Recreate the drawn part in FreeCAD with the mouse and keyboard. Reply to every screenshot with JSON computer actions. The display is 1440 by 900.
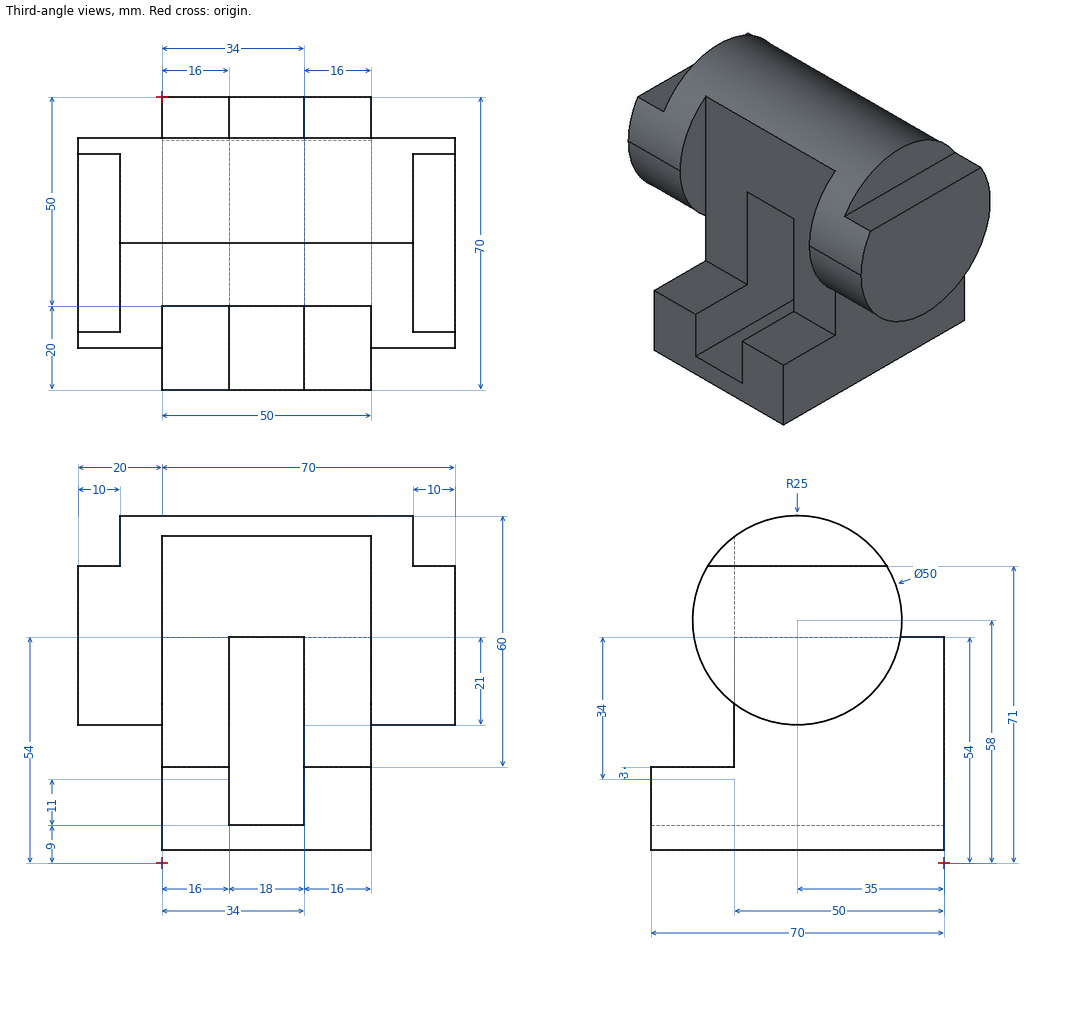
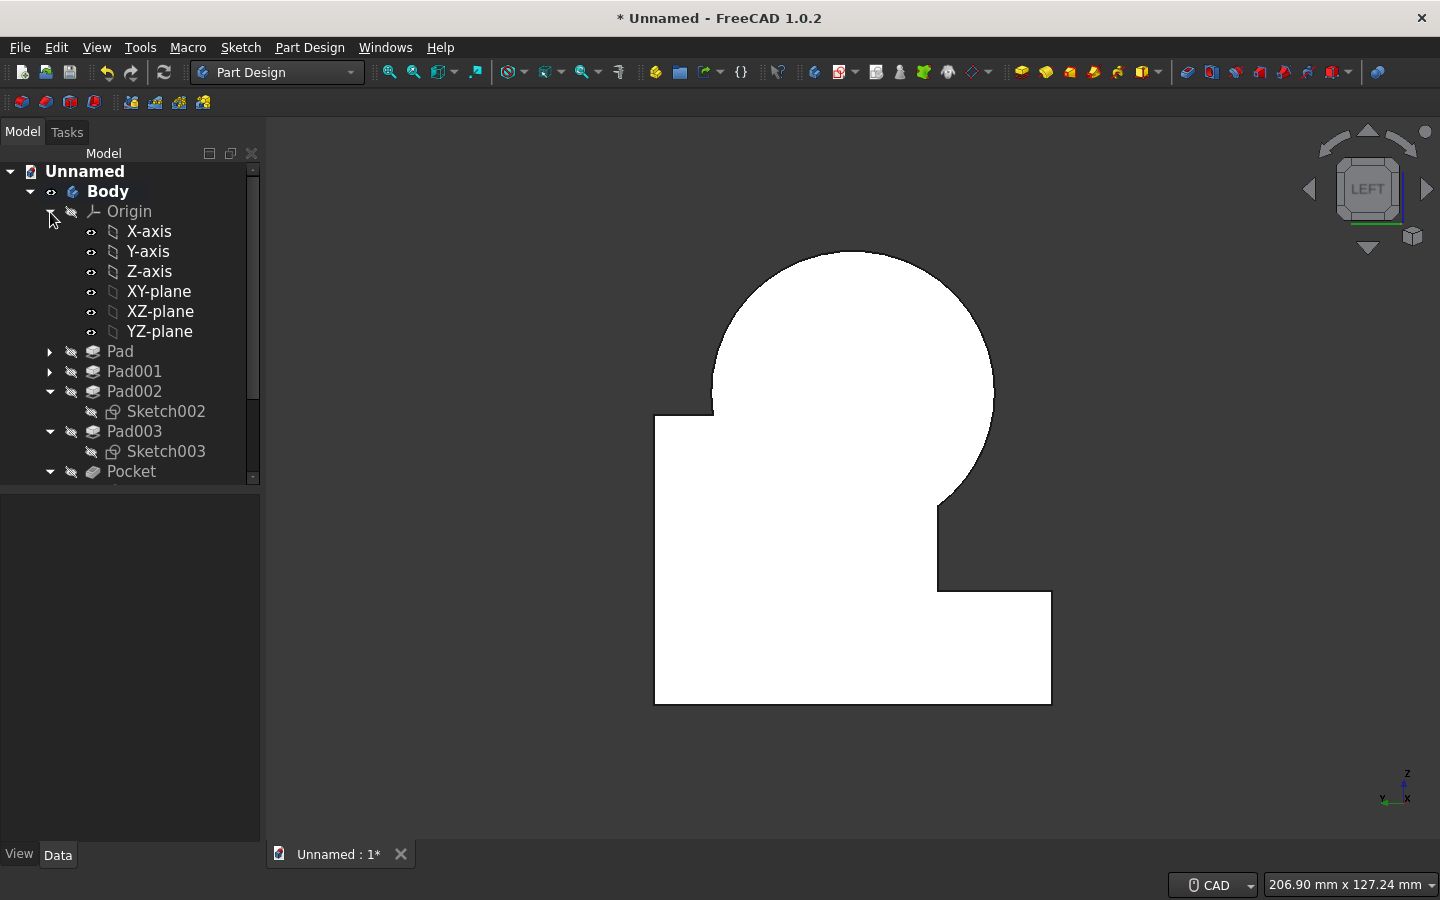
{"action": "left_click", "coordinate": [136, 332]}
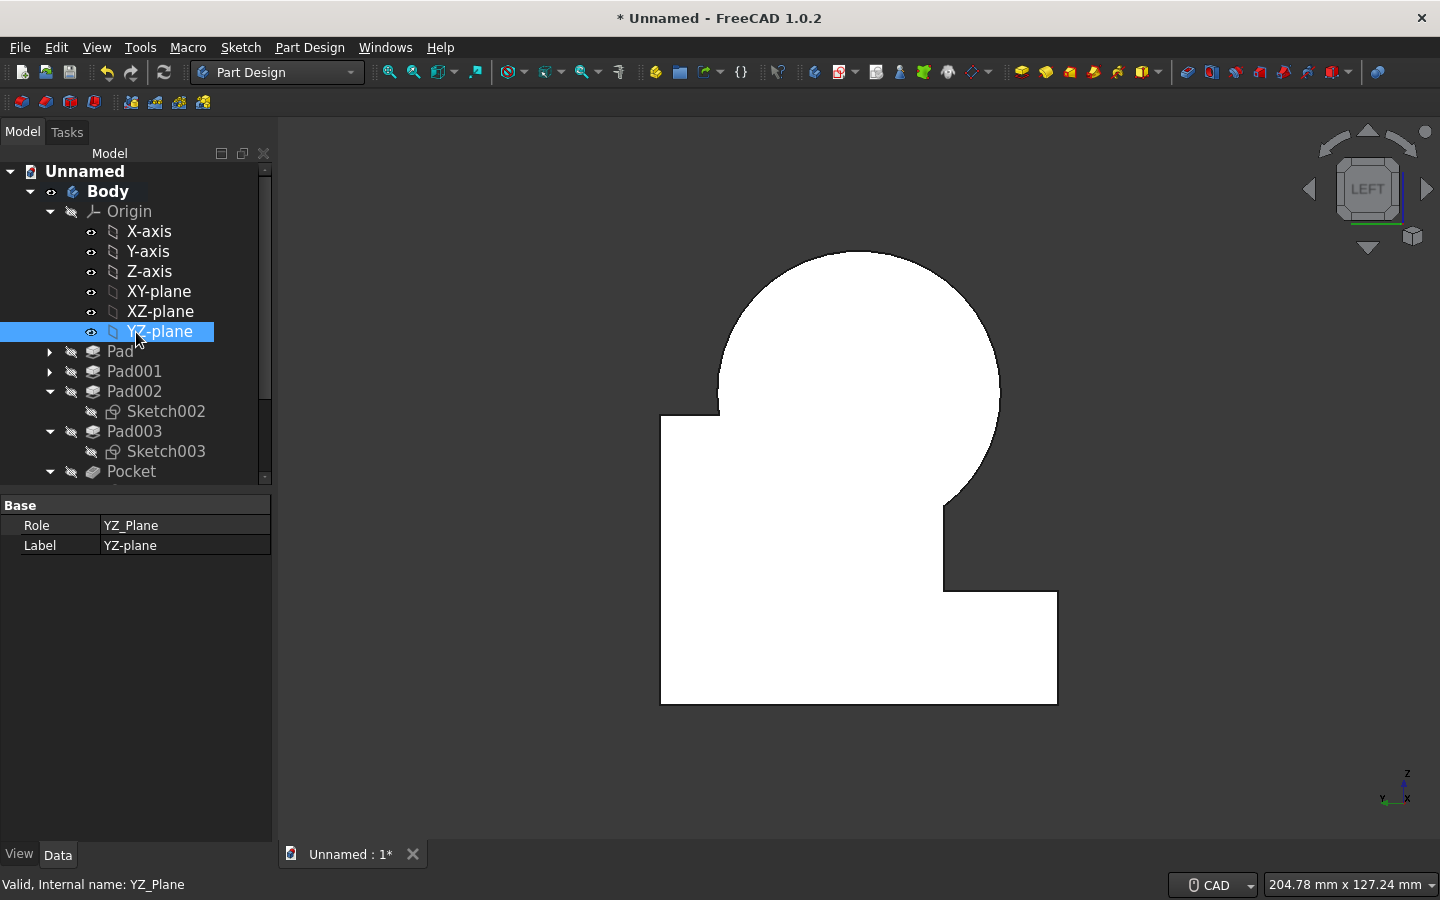
{"action": "left_click", "coordinate": [972, 72]}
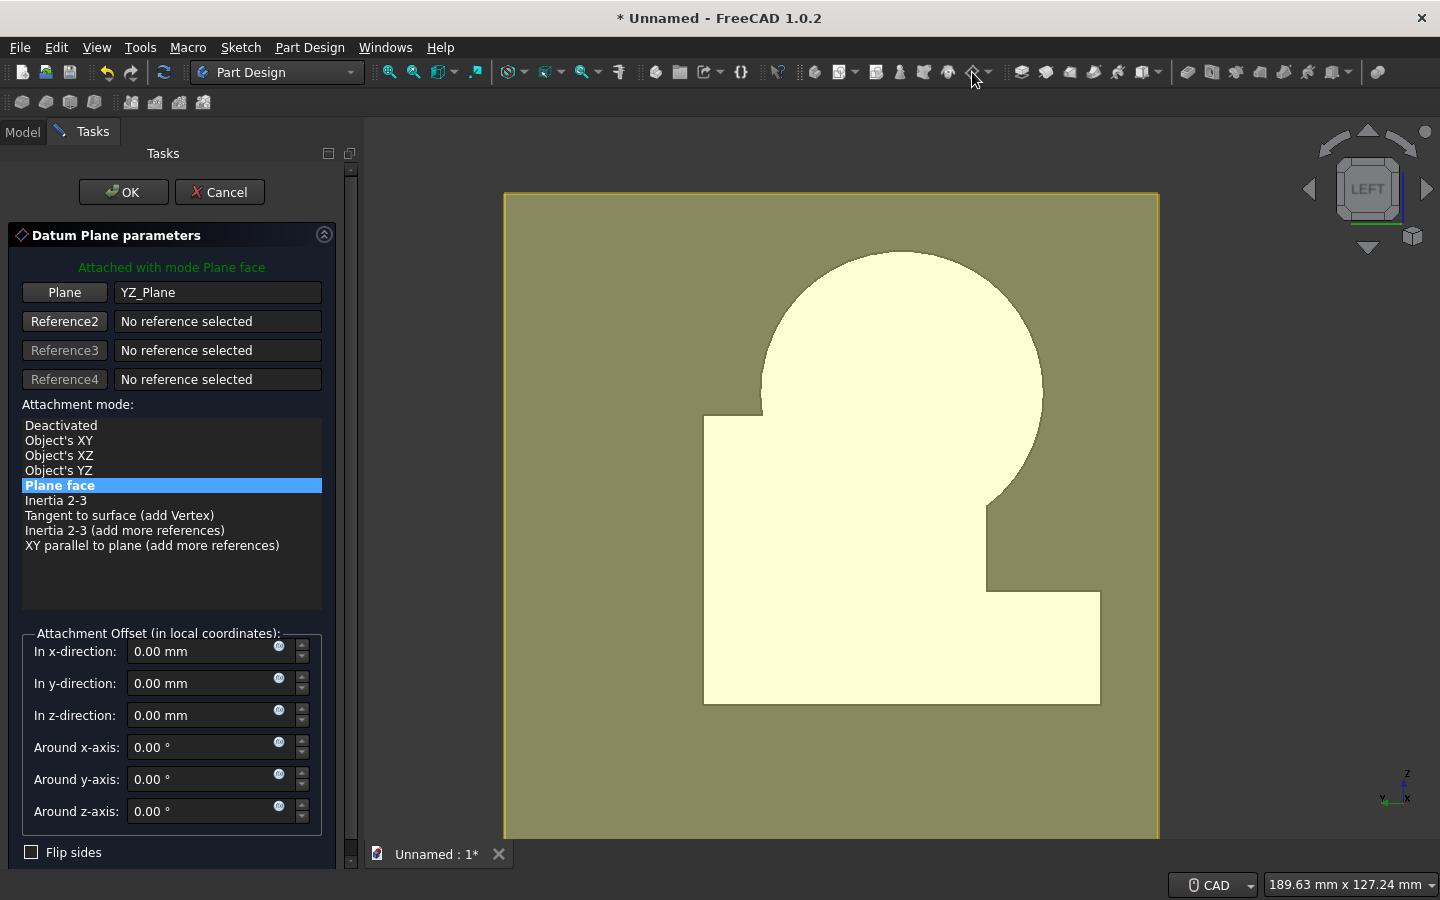
{"action": "triple_click", "coordinate": [210, 715]}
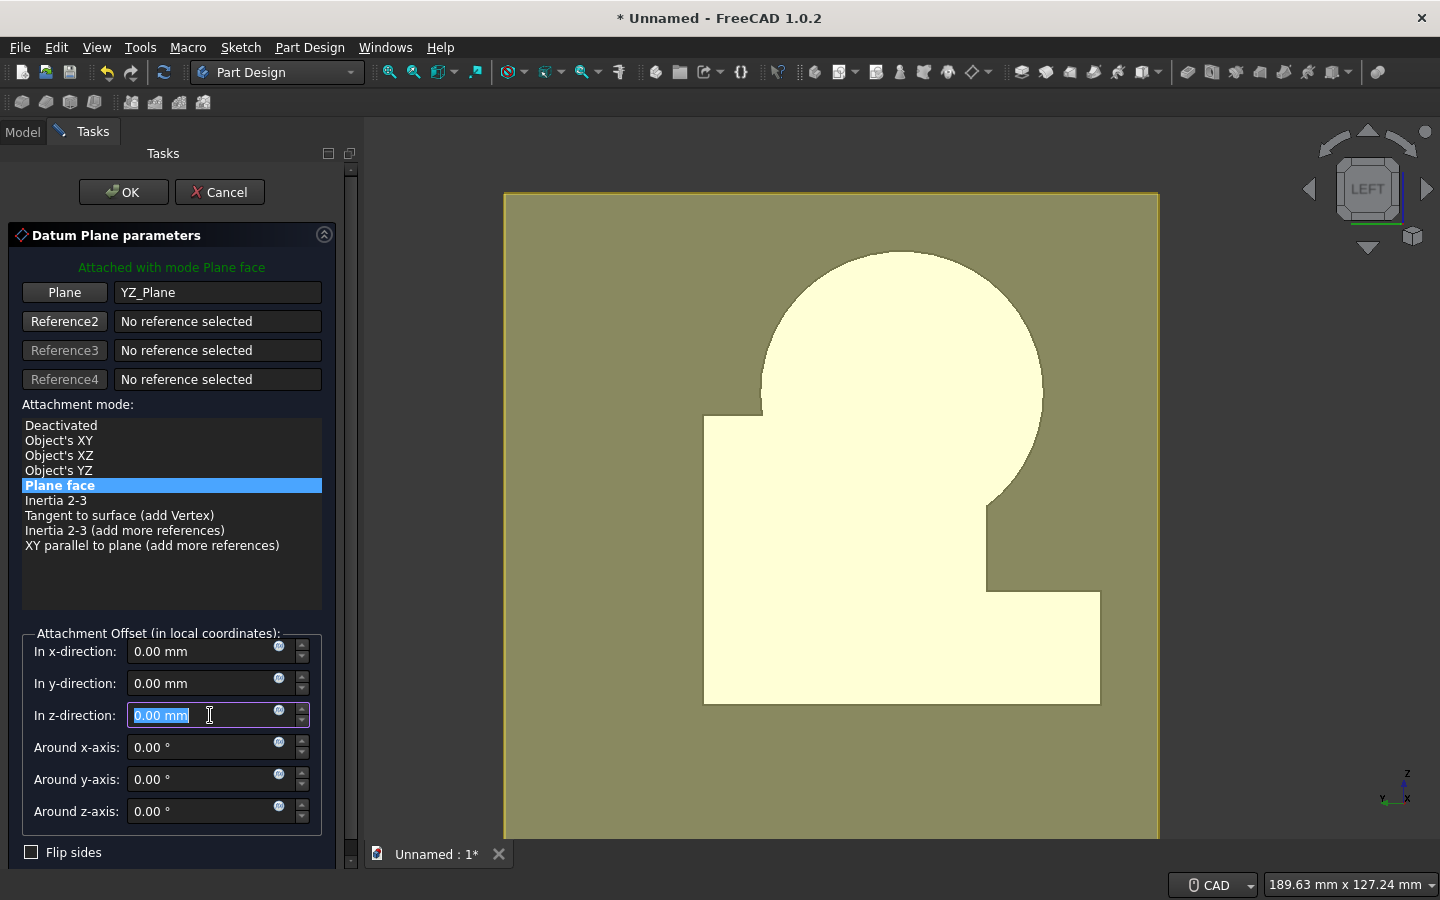
{"action": "type", "text": "-20"}
{"action": "key", "text": "Tab"}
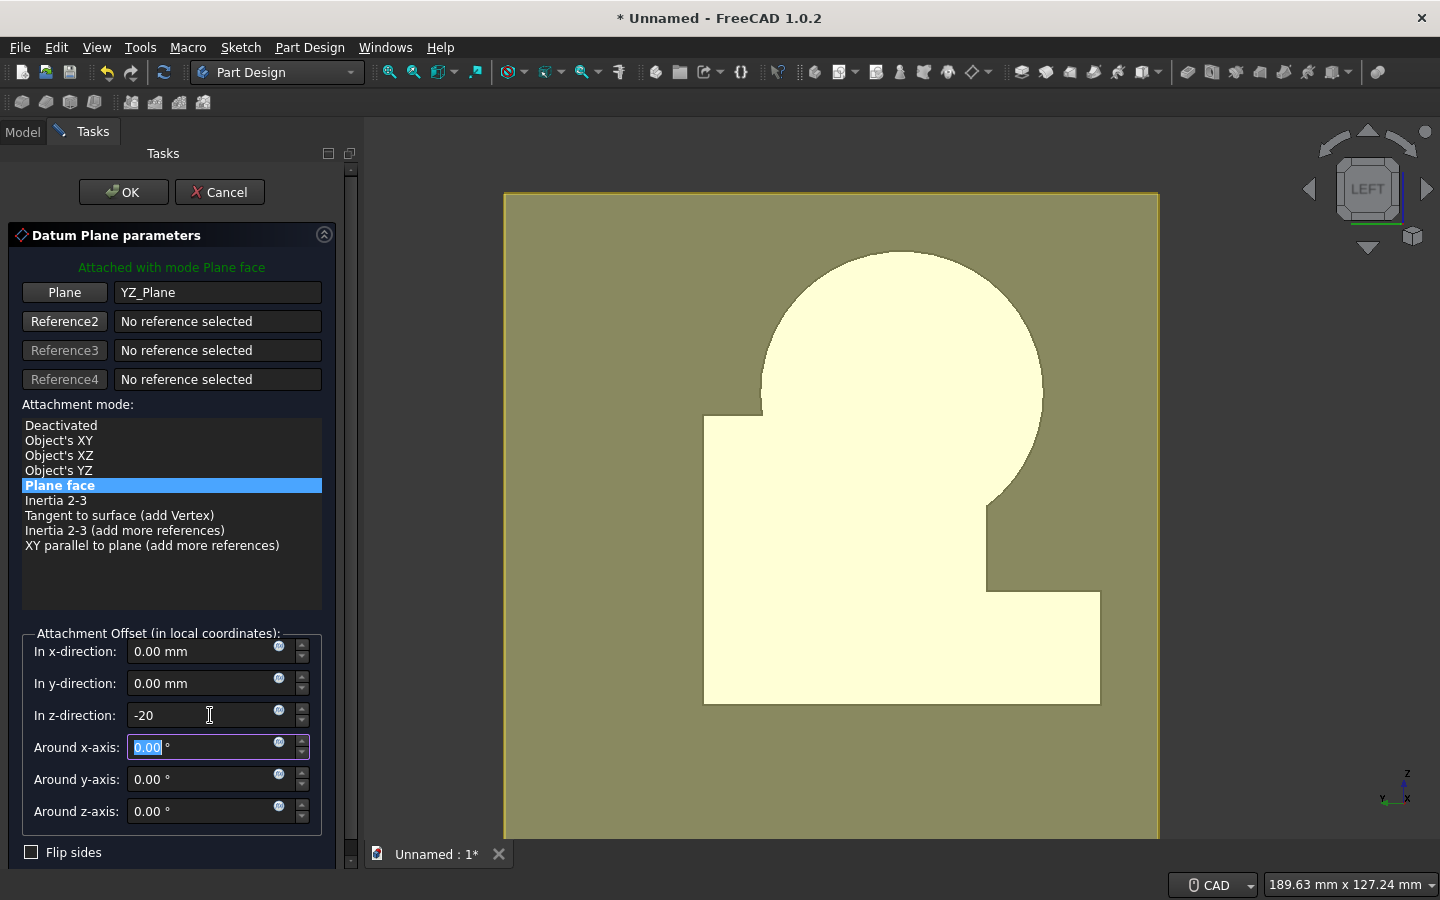
{"action": "left_click", "coordinate": [124, 192]}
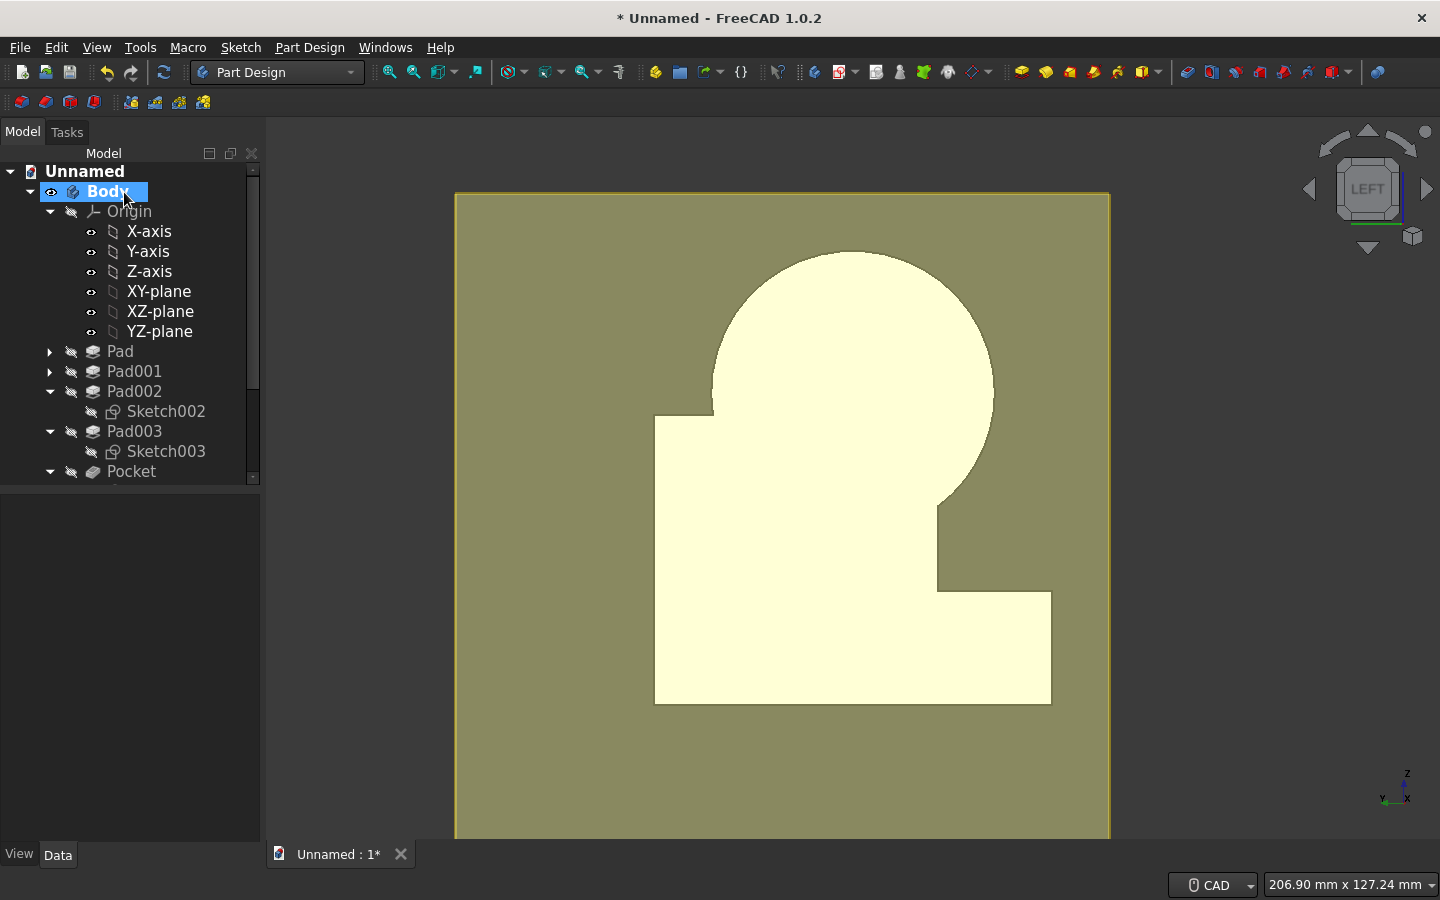
{"action": "scroll", "coordinate": [100, 327], "scroll_direction": "down", "scroll_amount": 3}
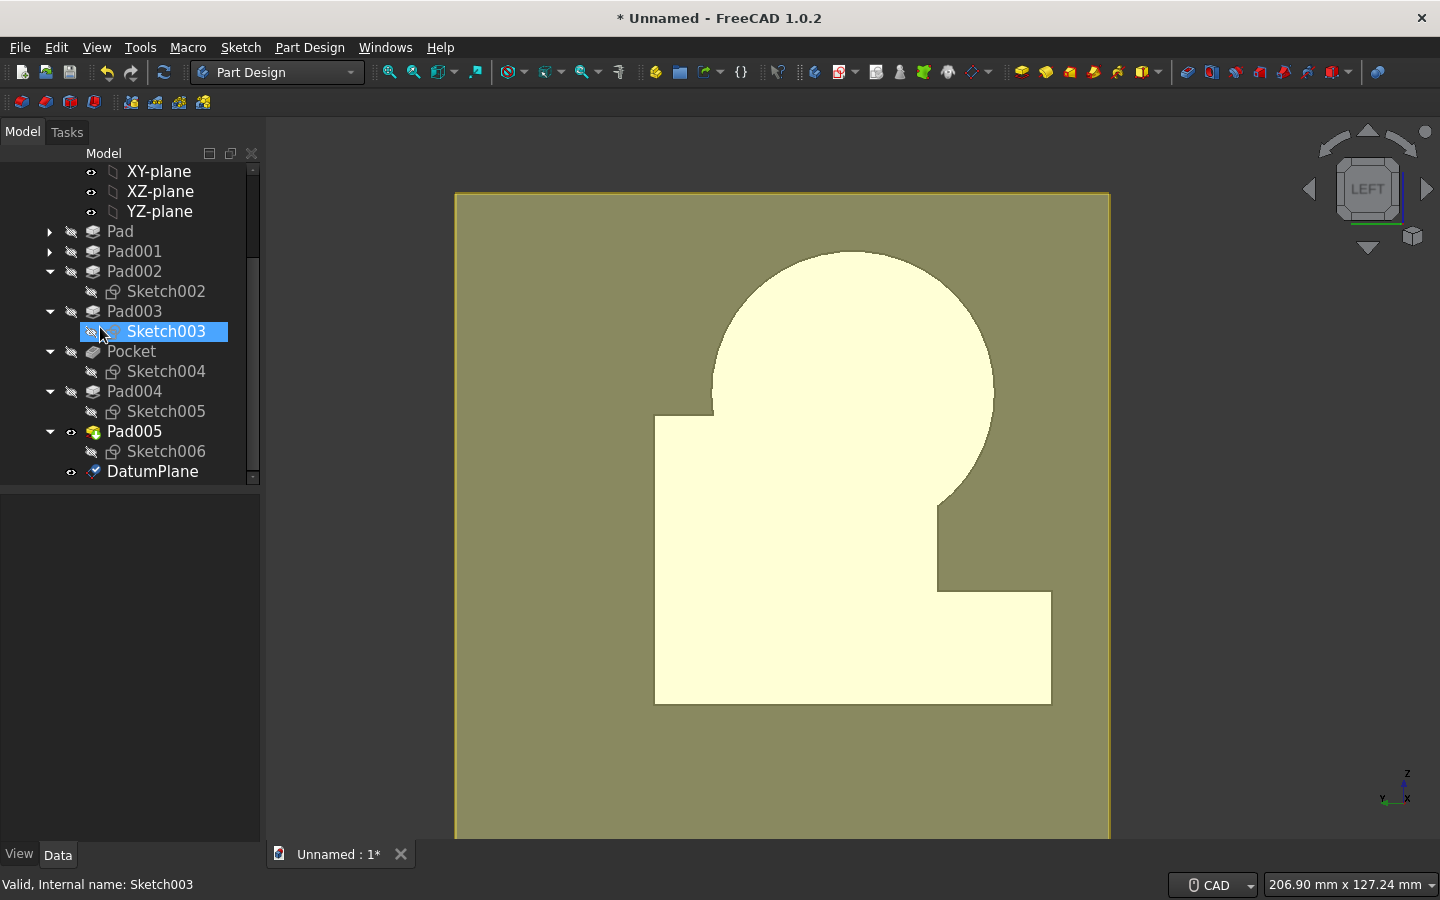
{"action": "left_click", "coordinate": [116, 472]}